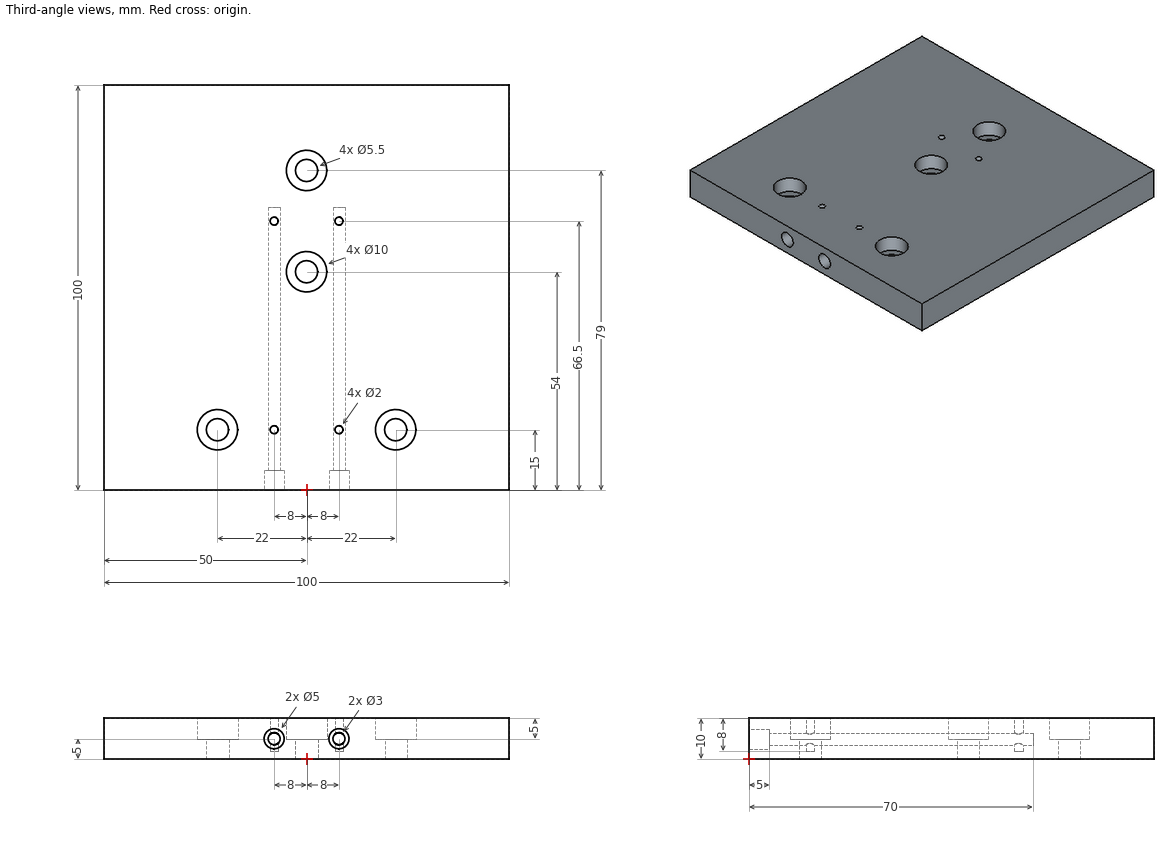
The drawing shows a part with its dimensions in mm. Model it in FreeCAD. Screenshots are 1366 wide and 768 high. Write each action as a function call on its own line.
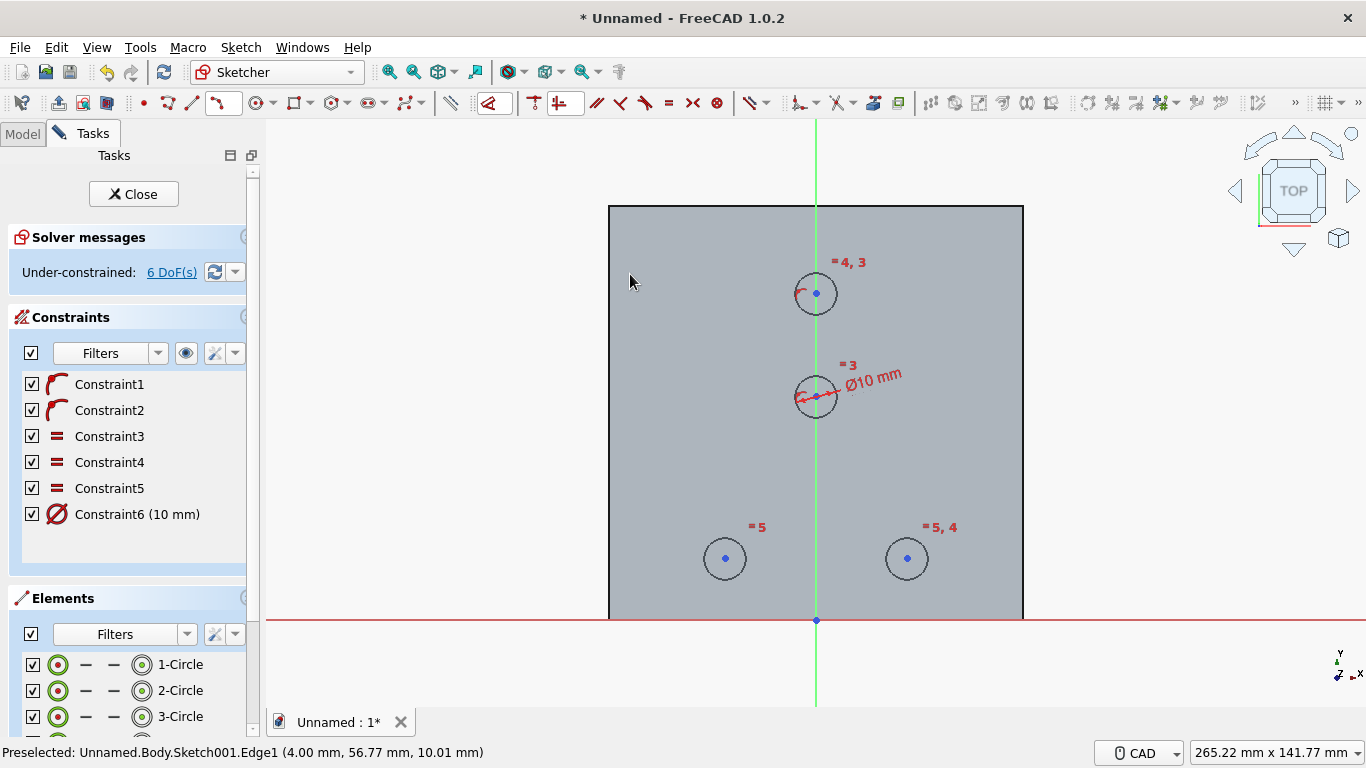
click(816, 397)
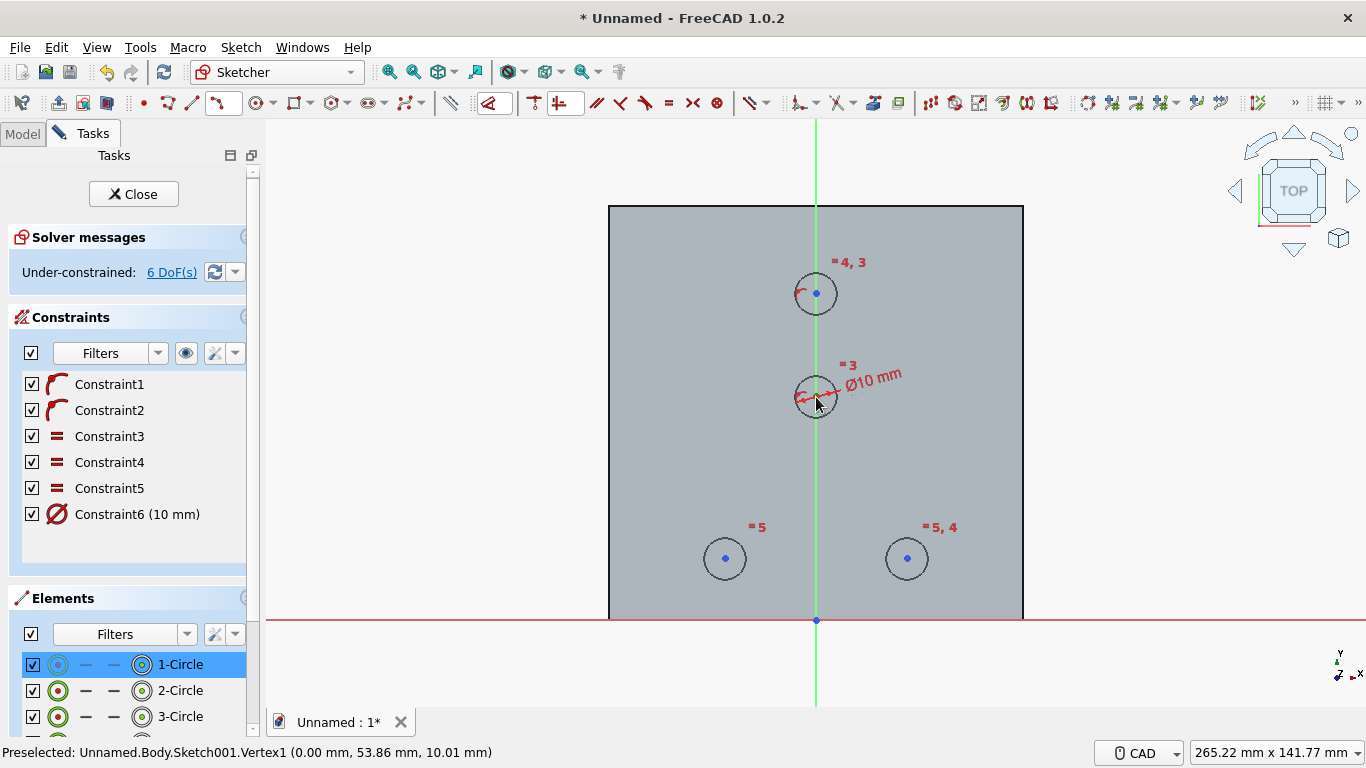
click(506, 104)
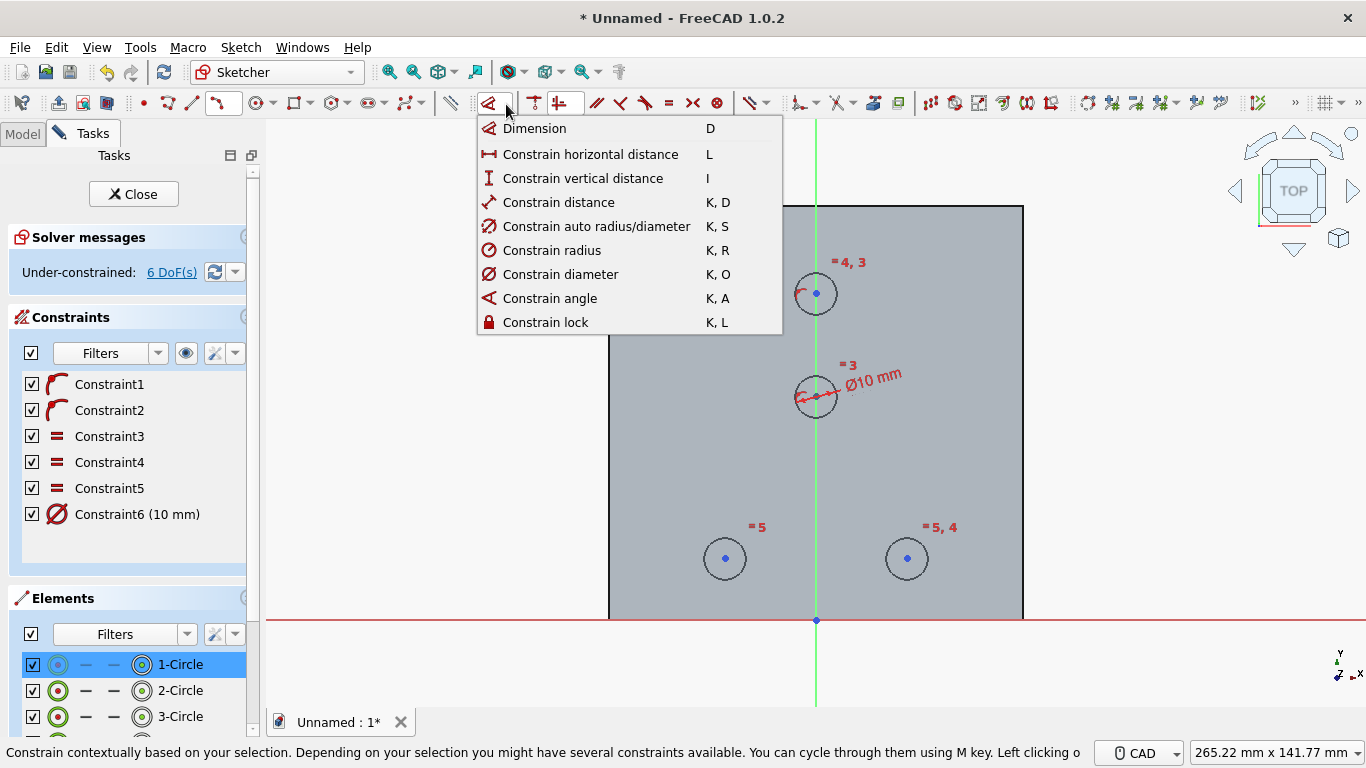
click(630, 178)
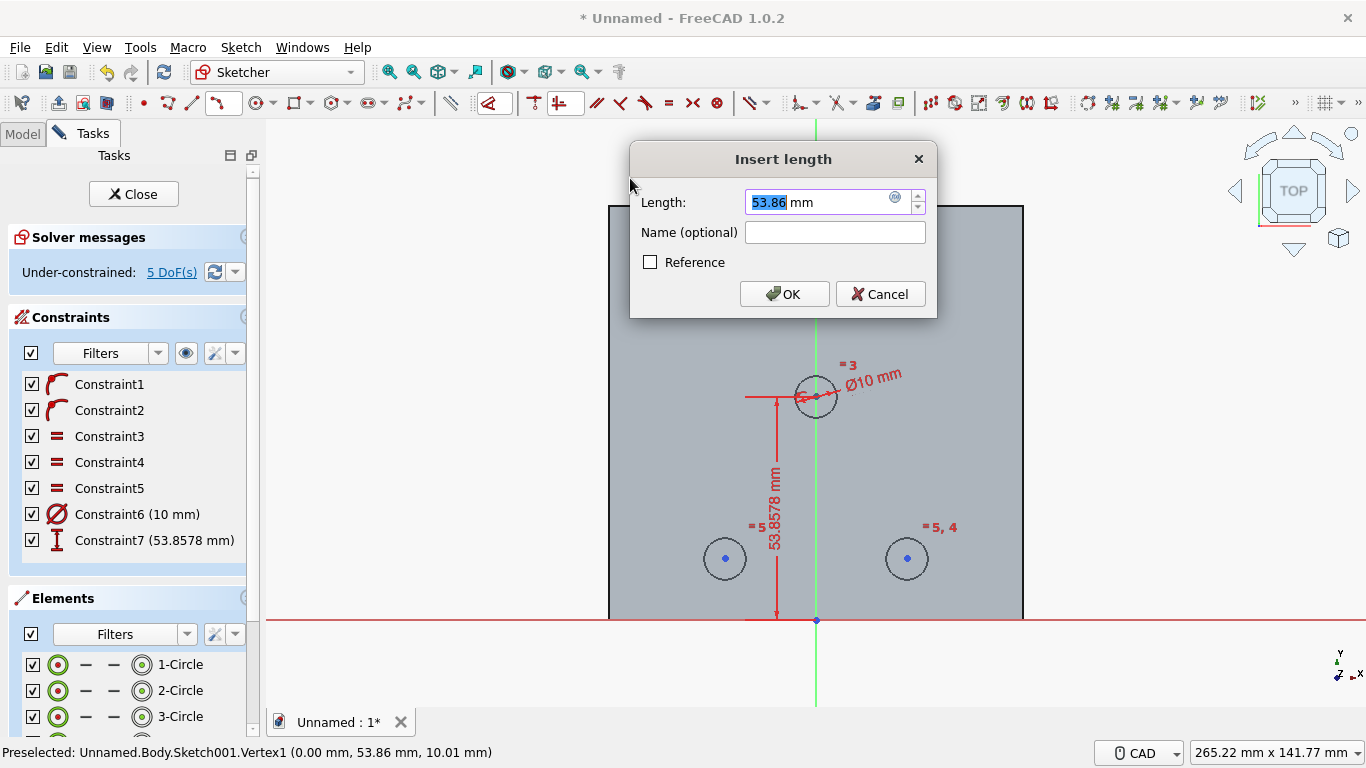
text(54)
key(Return)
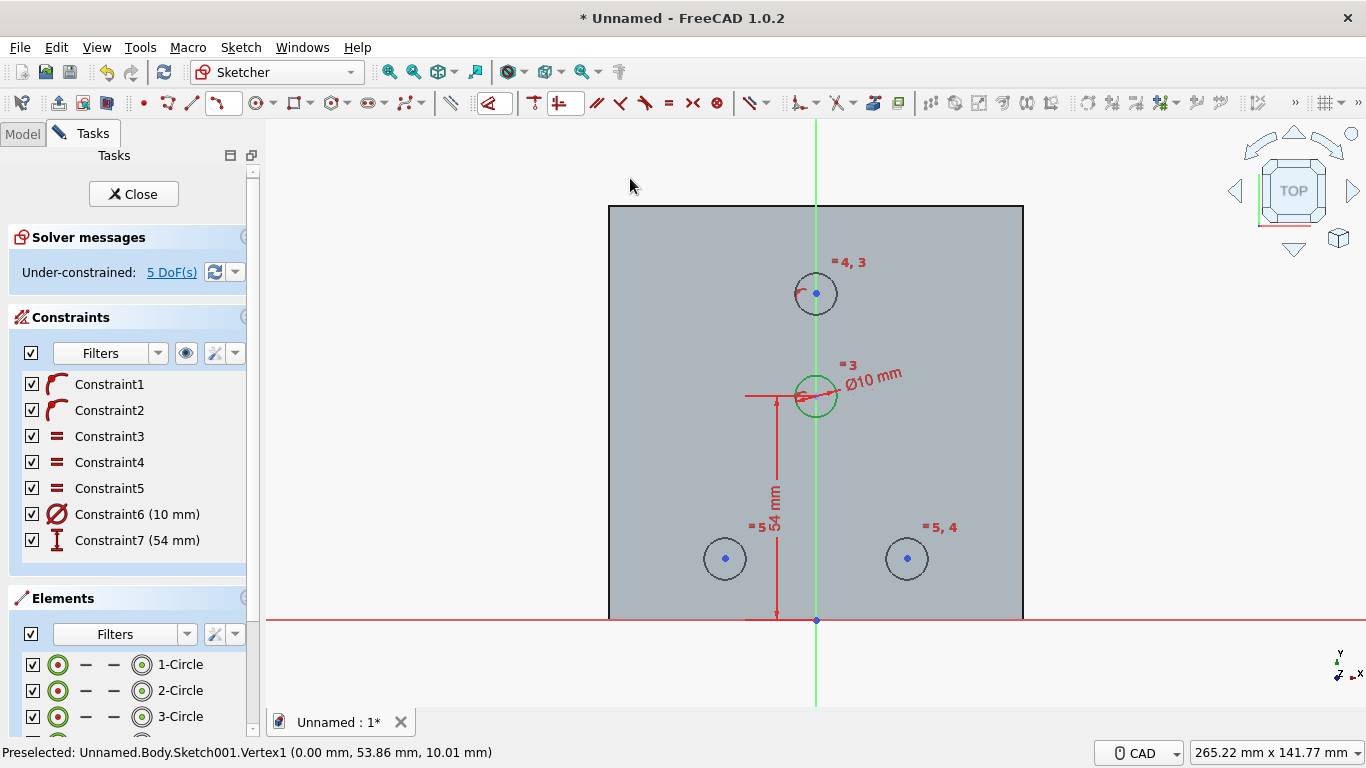
click(816, 294)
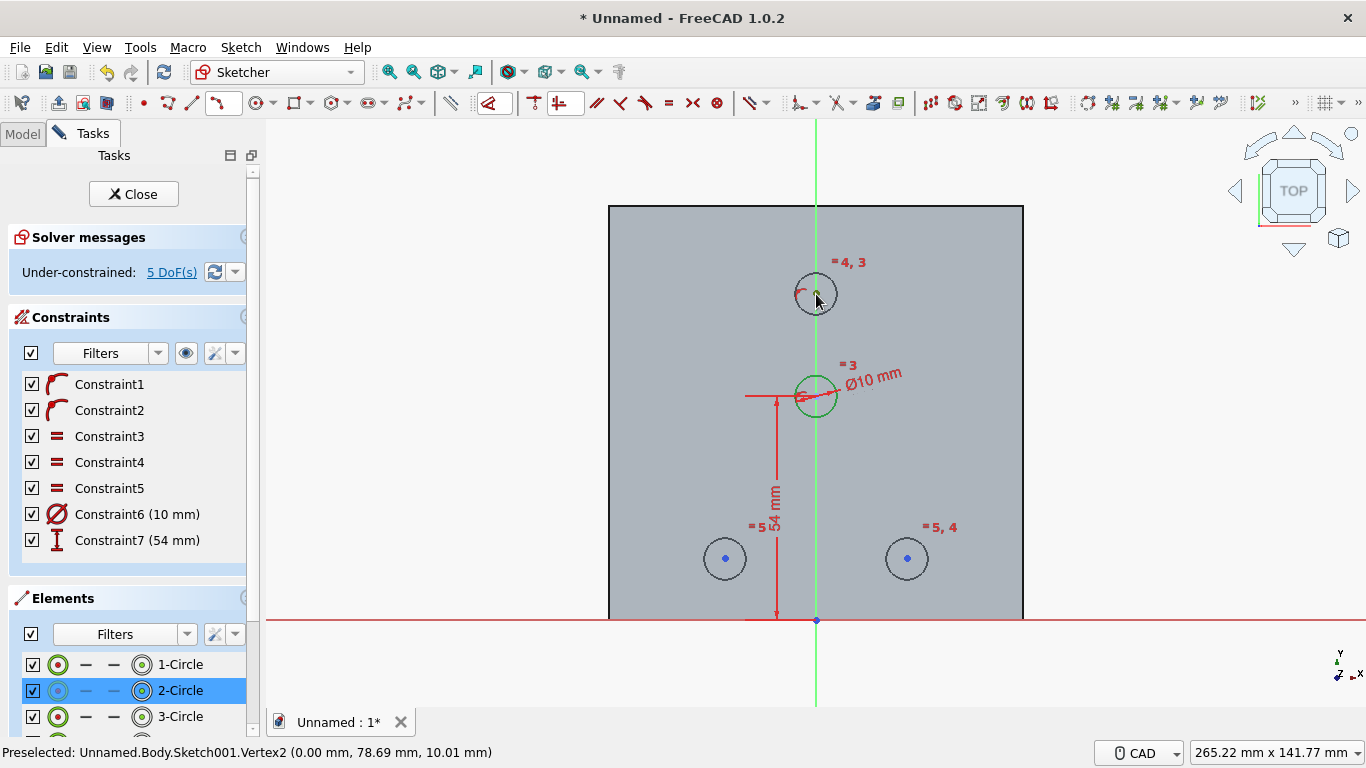
click(506, 104)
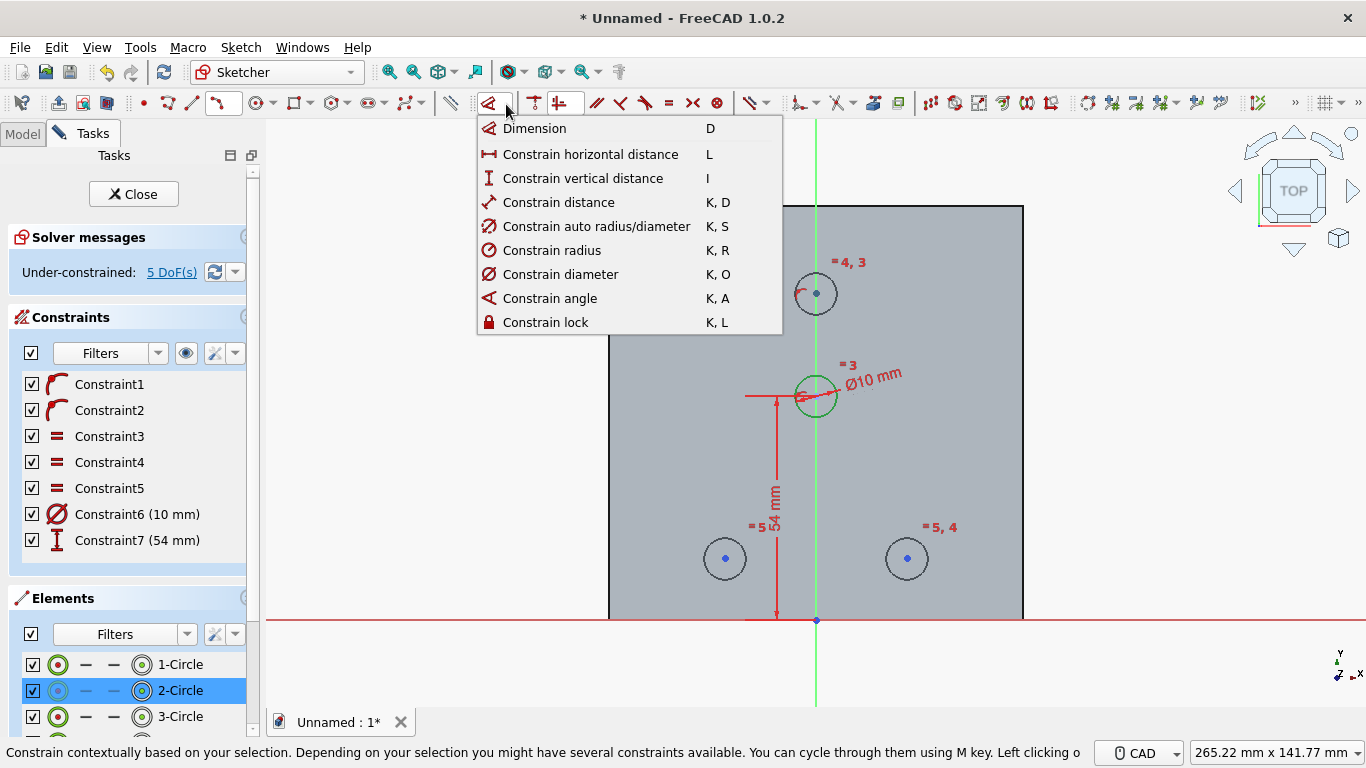
click(630, 178)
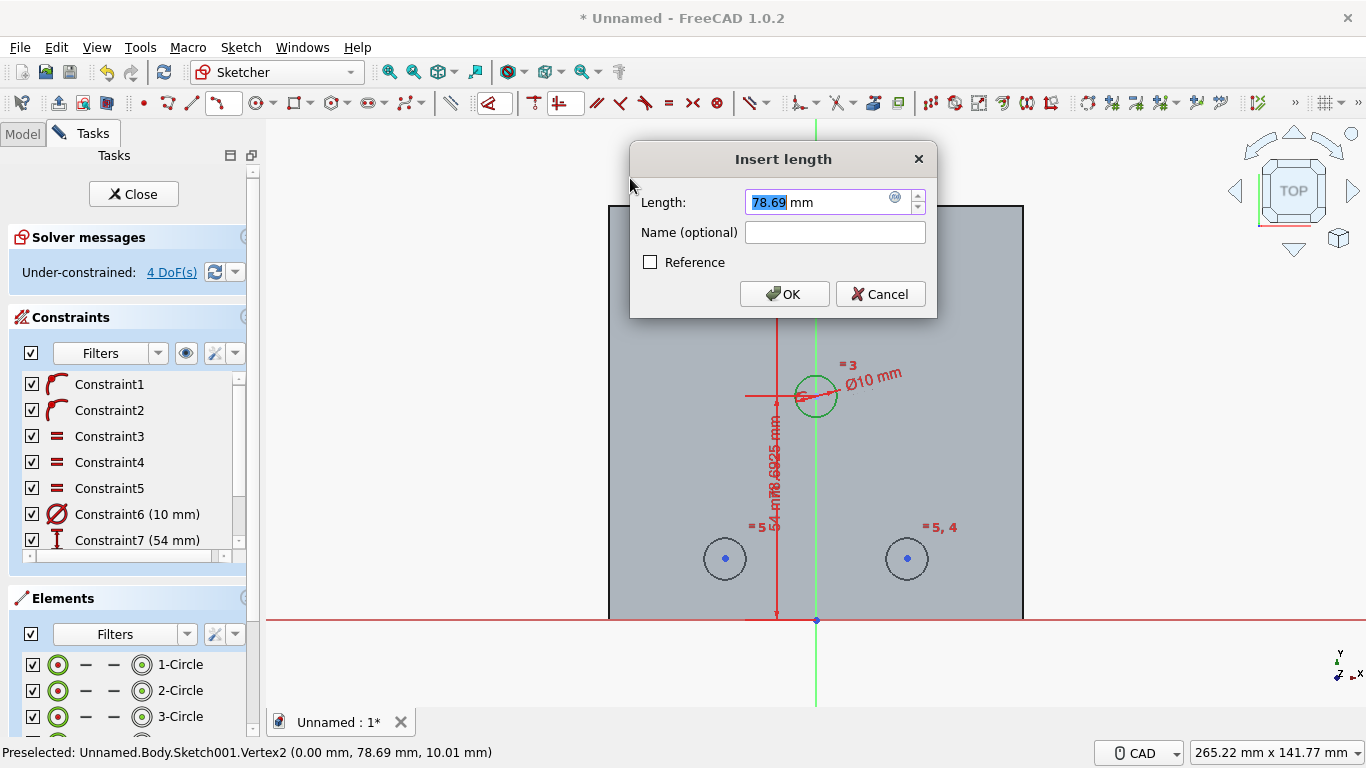
text(79)
key(Return)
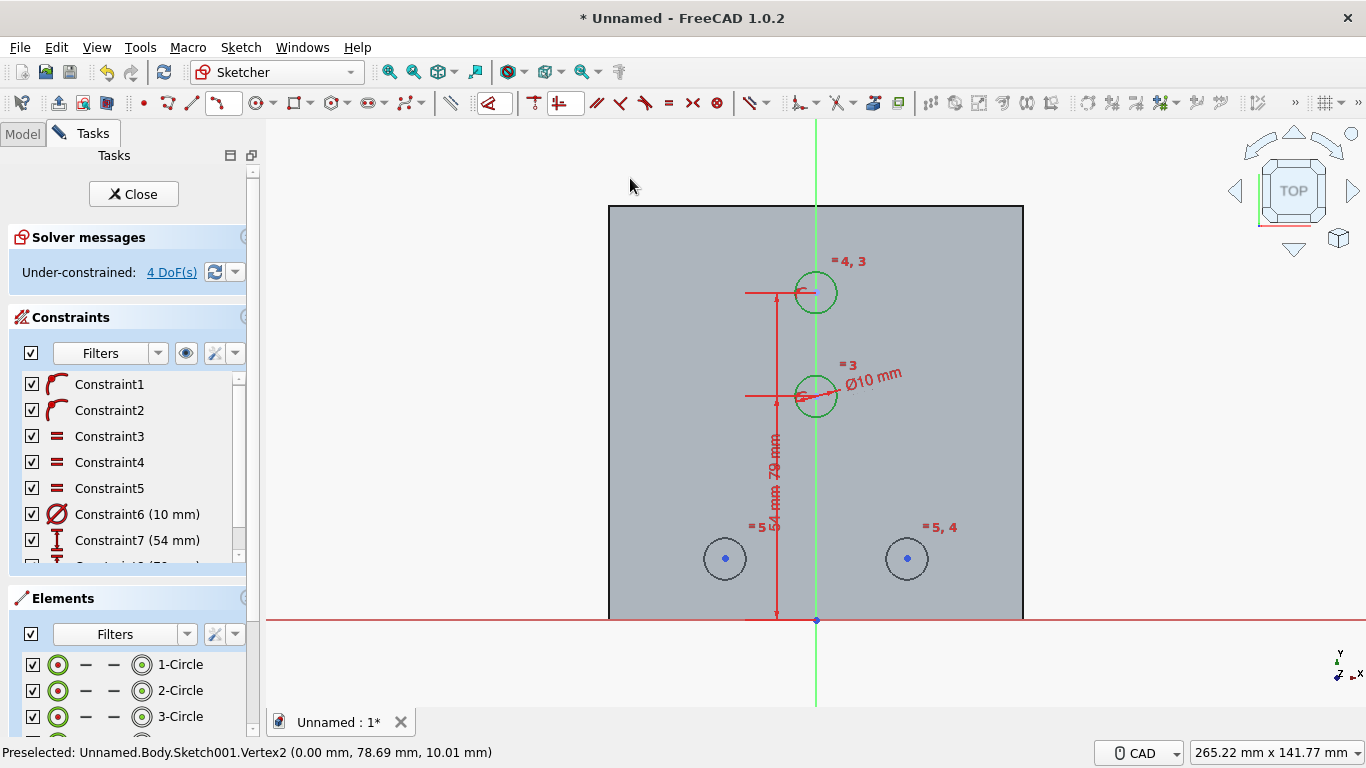
click(907, 559)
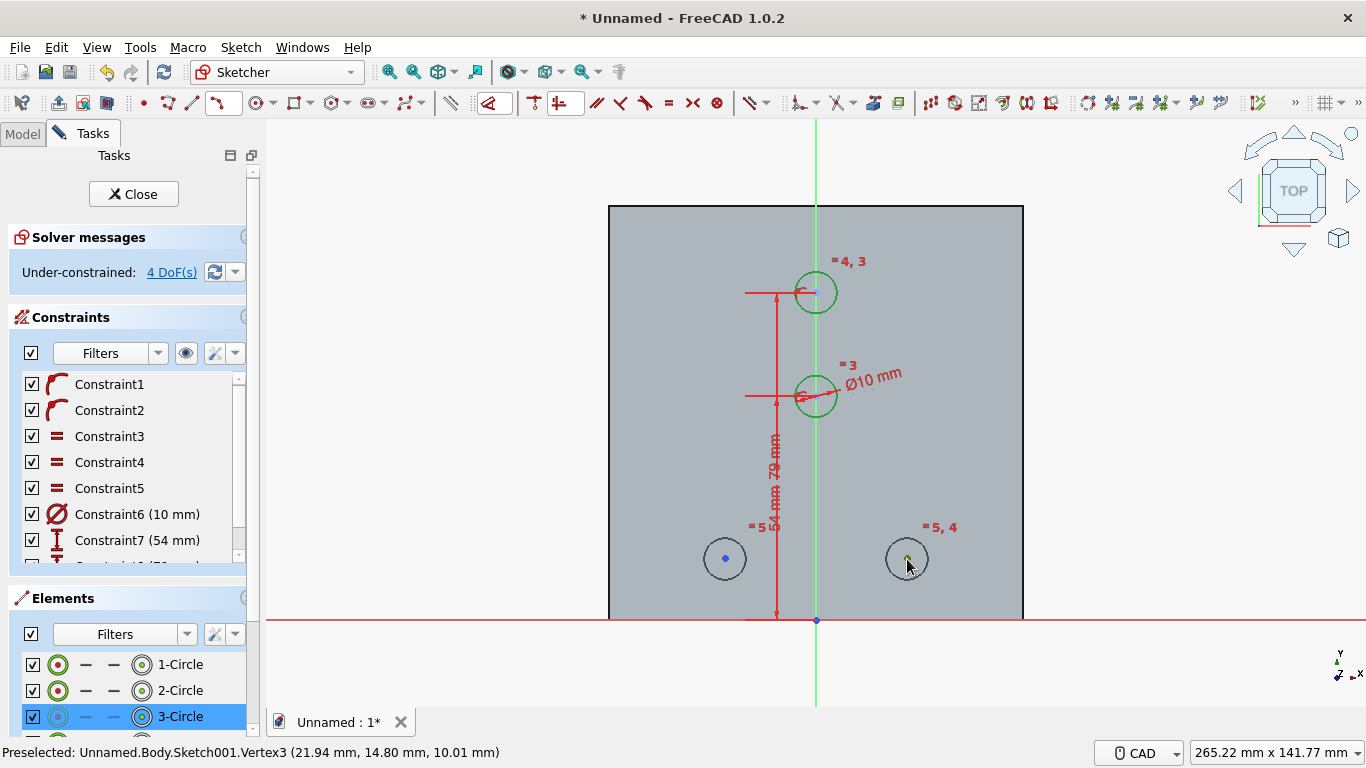
key(l)